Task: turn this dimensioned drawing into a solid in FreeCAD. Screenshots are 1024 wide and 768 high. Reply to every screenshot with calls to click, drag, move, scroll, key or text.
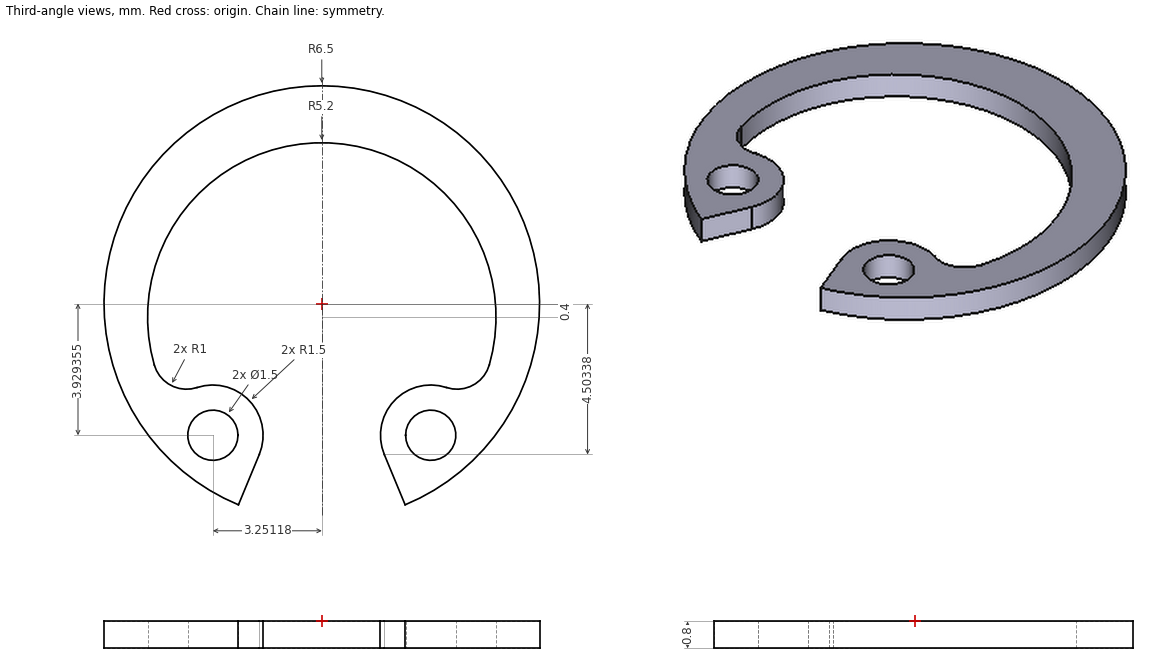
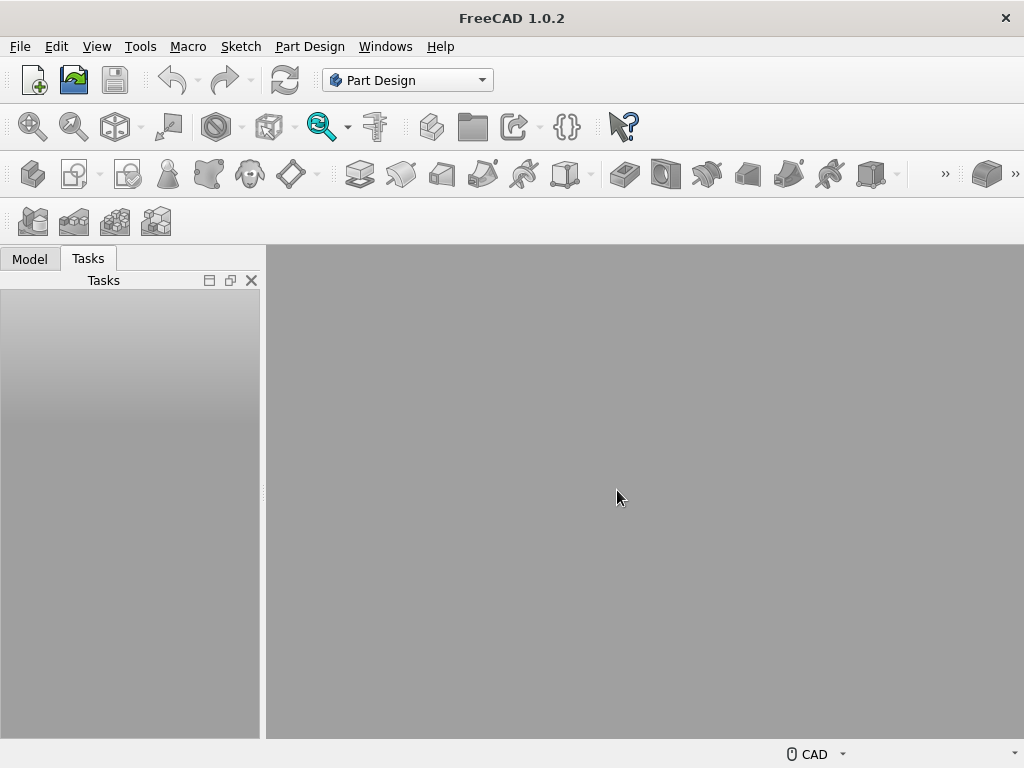
key(ctrl+n)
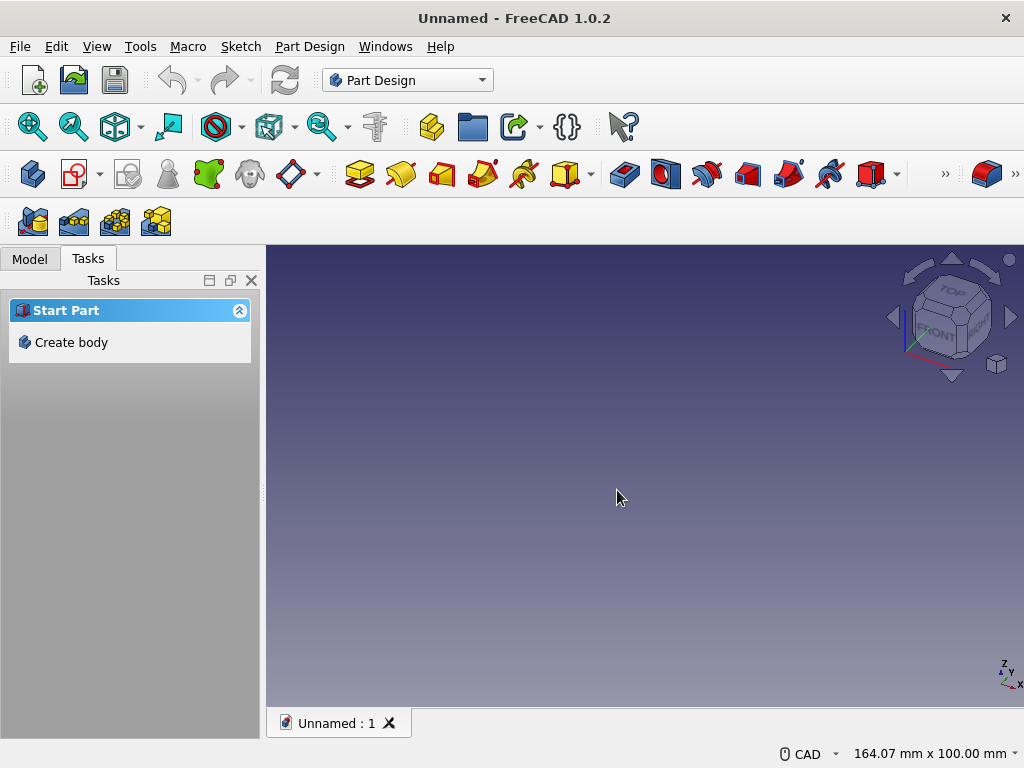
click(74, 174)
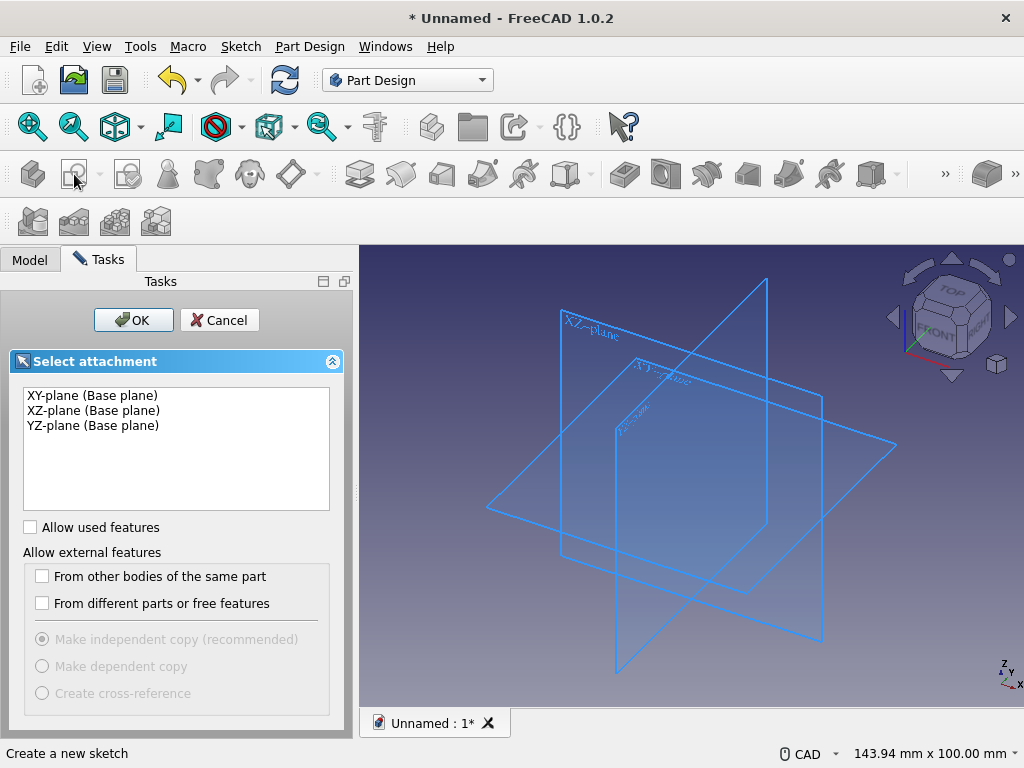
click(84, 396)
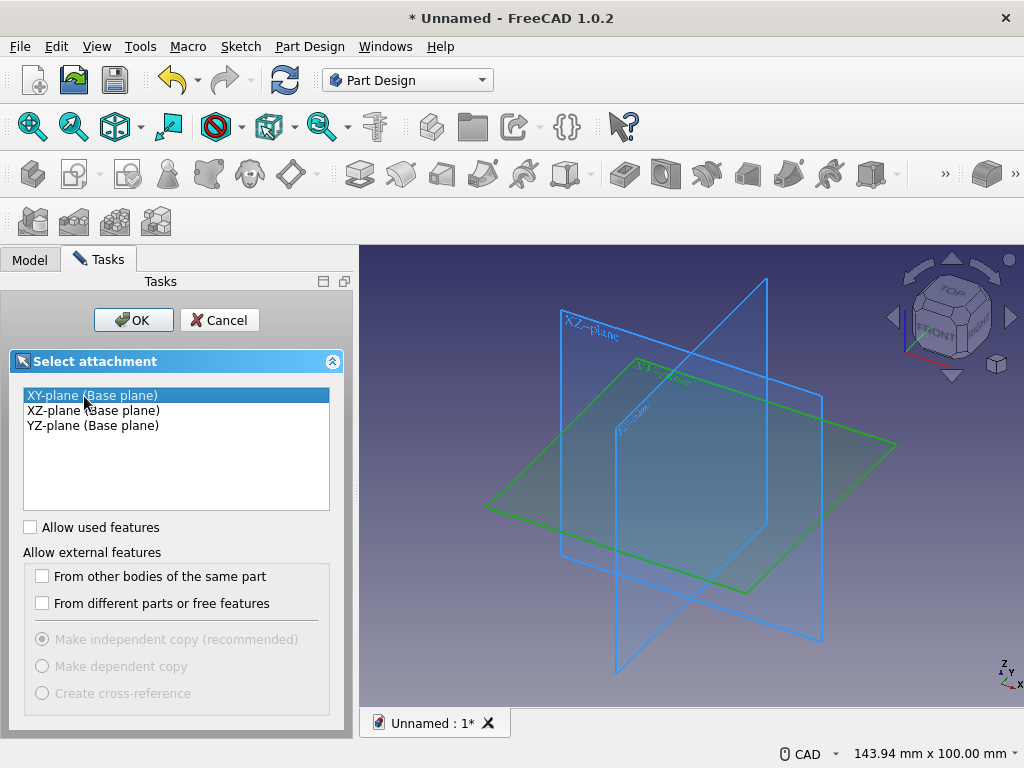
click(134, 320)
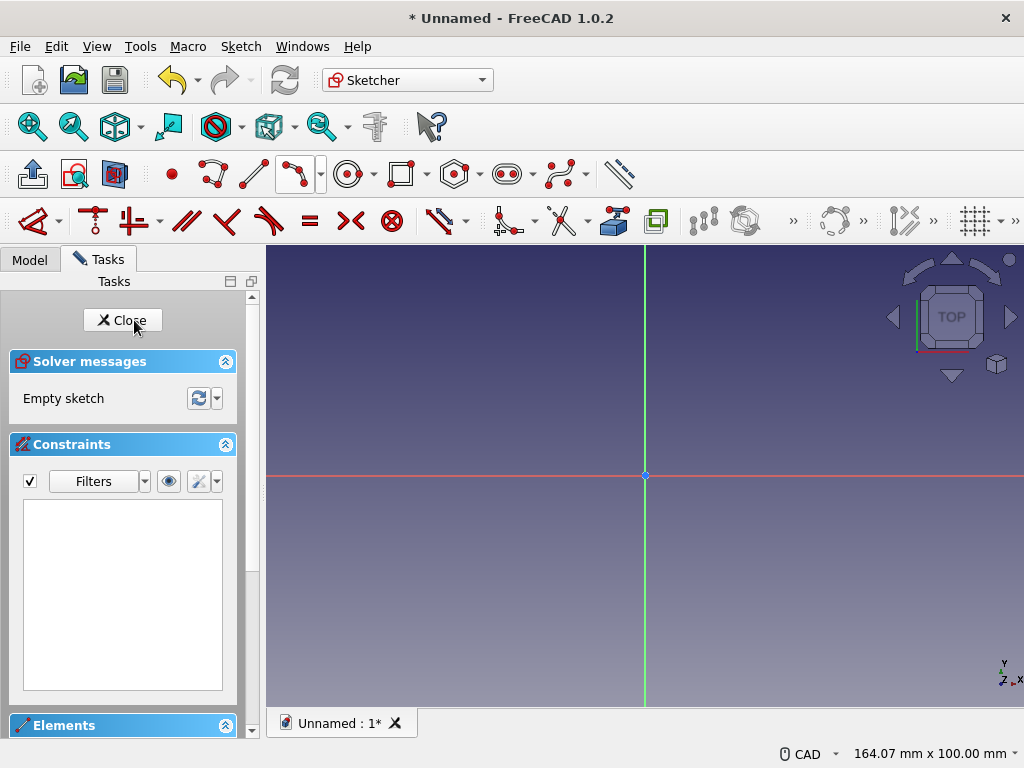
scroll(662, 475, up, 8)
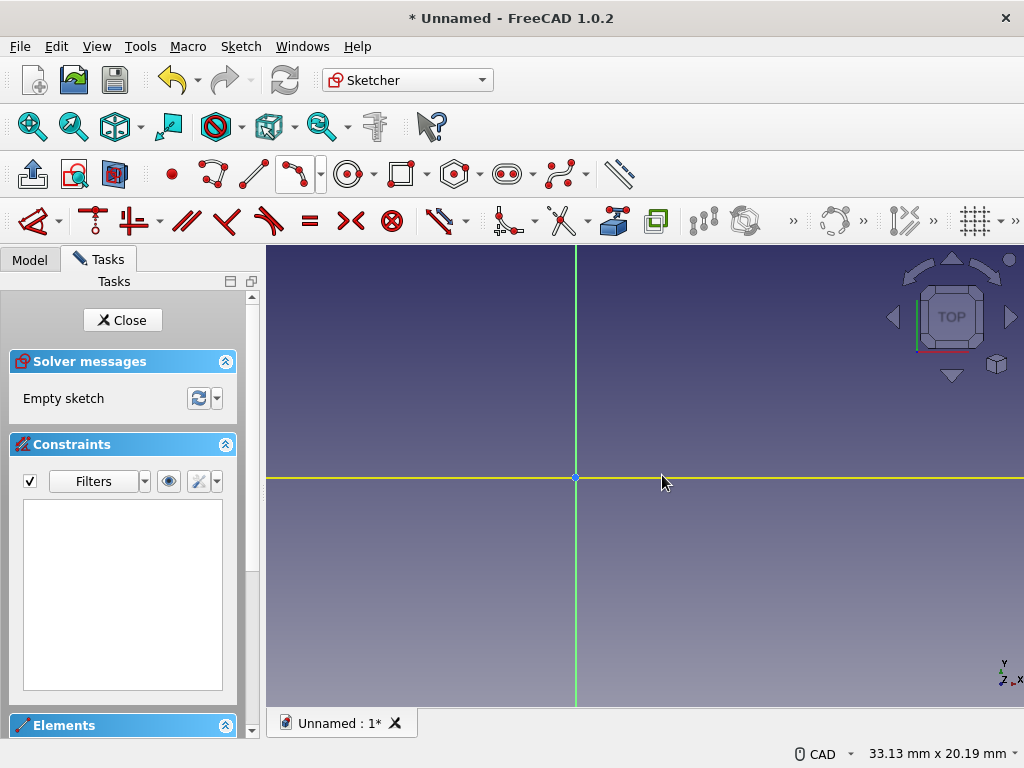
key(g)
key(l)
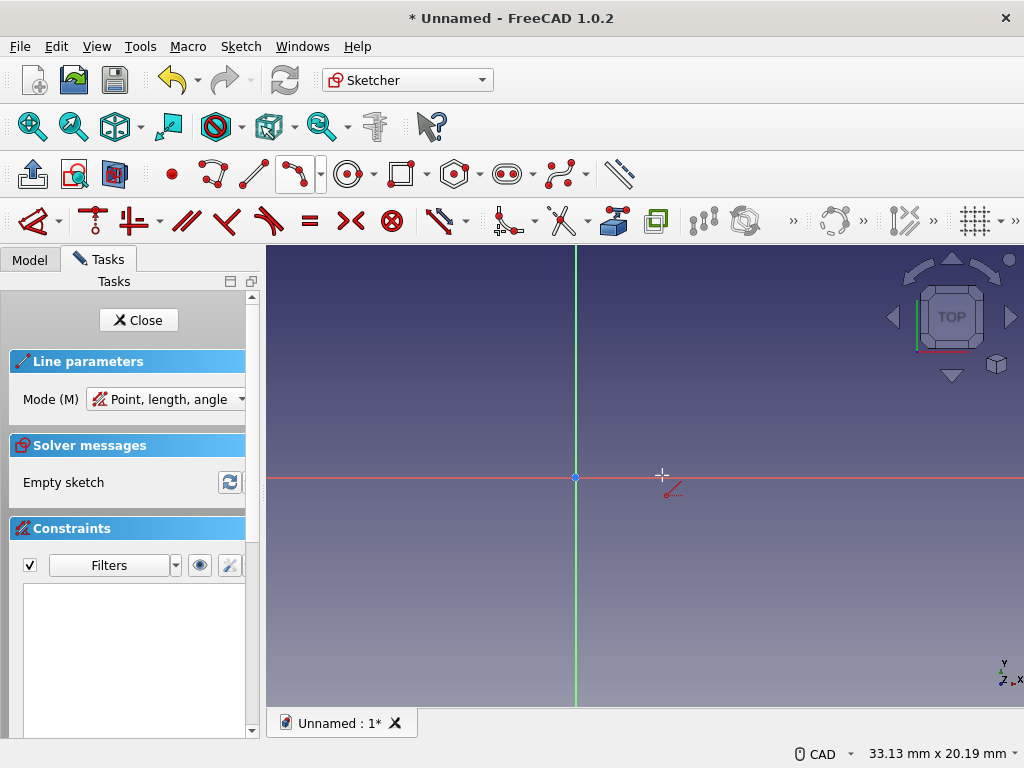
click(618, 581)
click(633, 615)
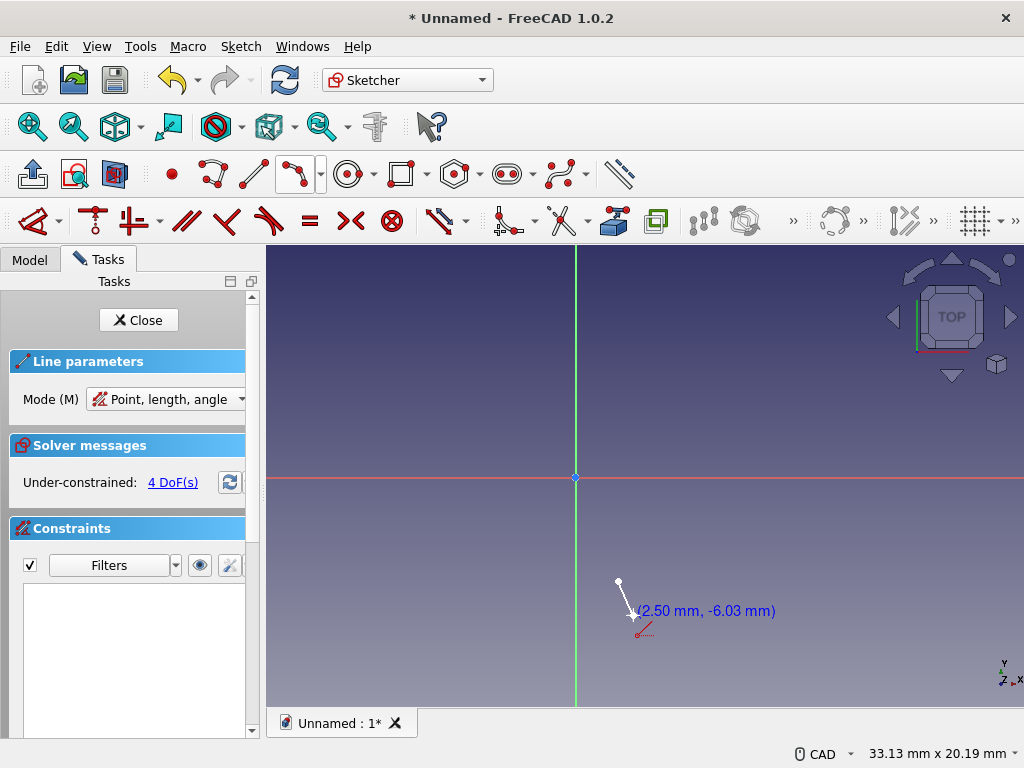
click(519, 615)
click(533, 581)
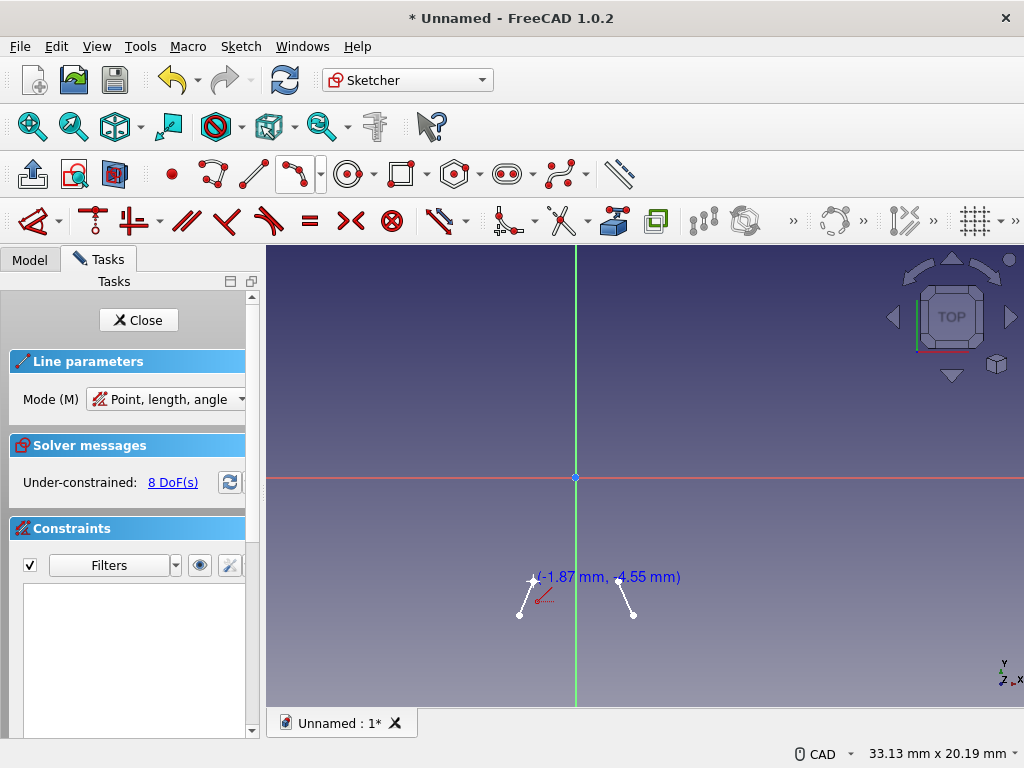
key(g)
key(3)
key(a)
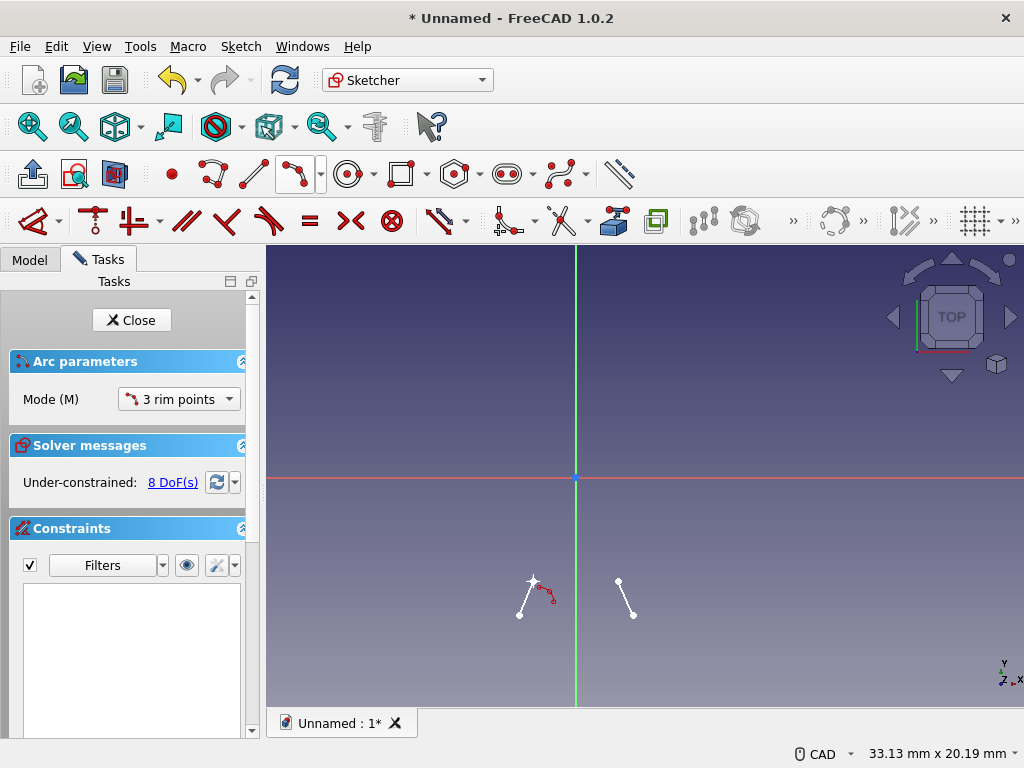
click(633, 616)
click(519, 616)
click(653, 351)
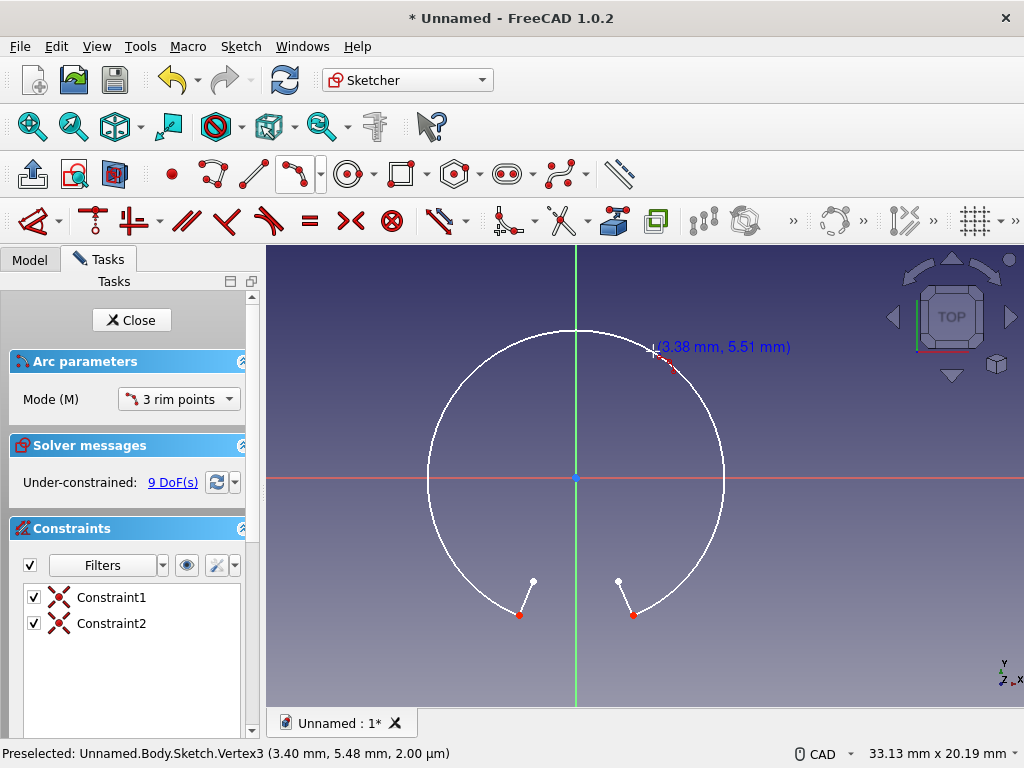
click(533, 582)
click(491, 535)
click(526, 545)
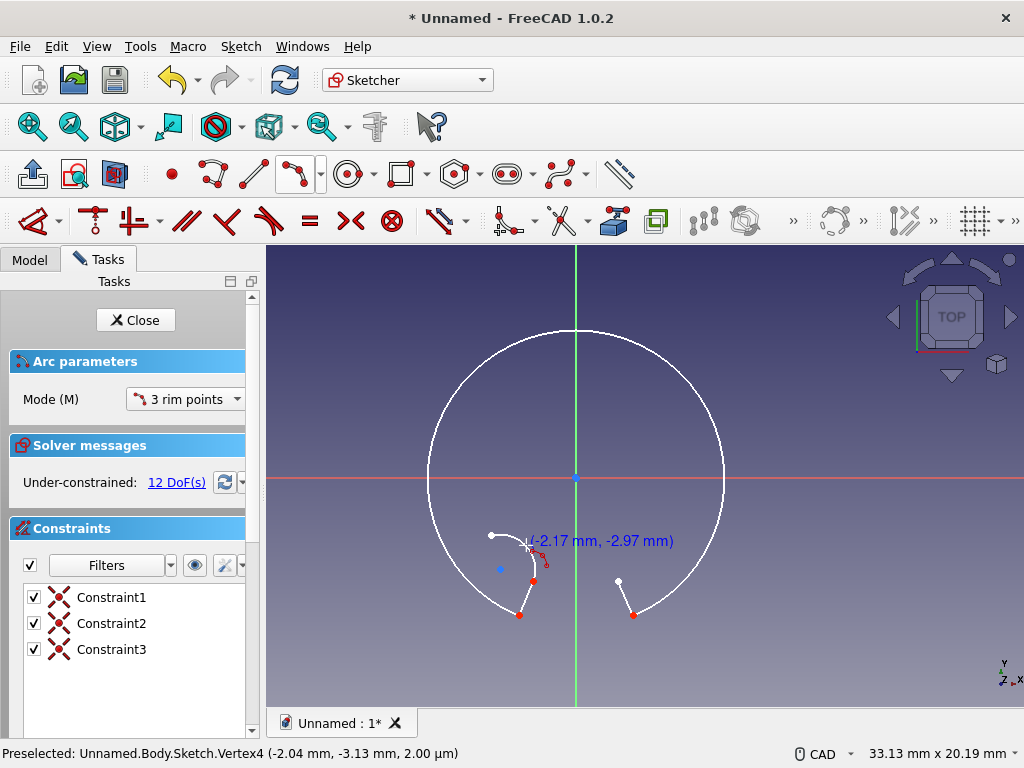
click(491, 536)
click(461, 520)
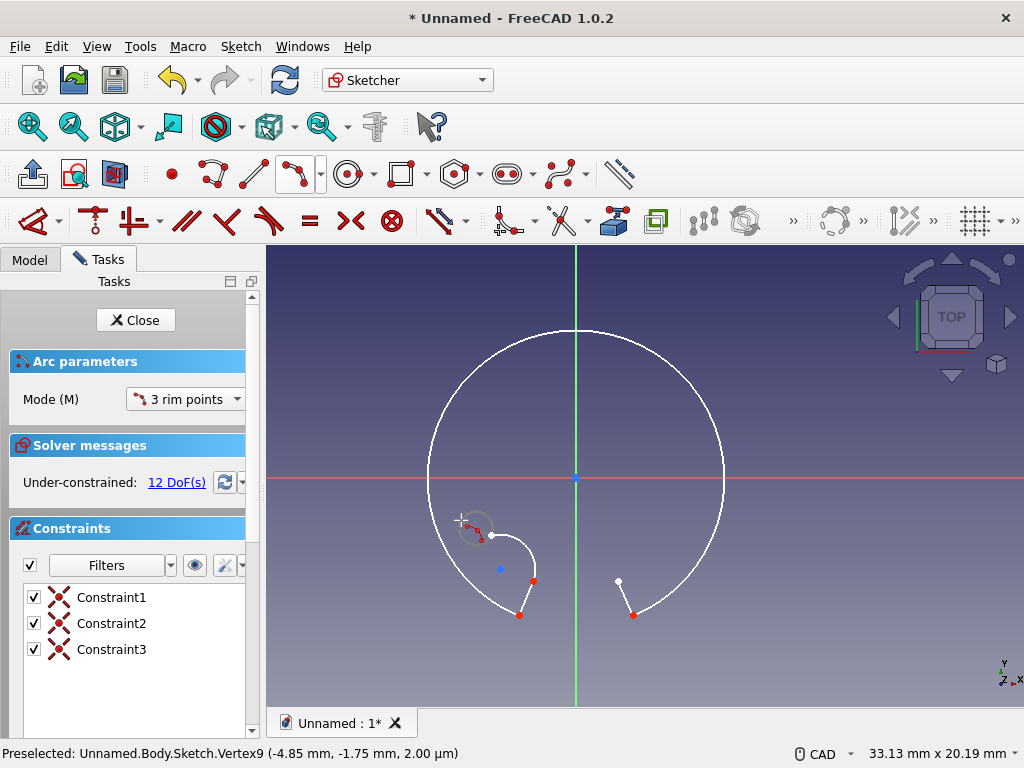
scroll(473, 534, up, 5)